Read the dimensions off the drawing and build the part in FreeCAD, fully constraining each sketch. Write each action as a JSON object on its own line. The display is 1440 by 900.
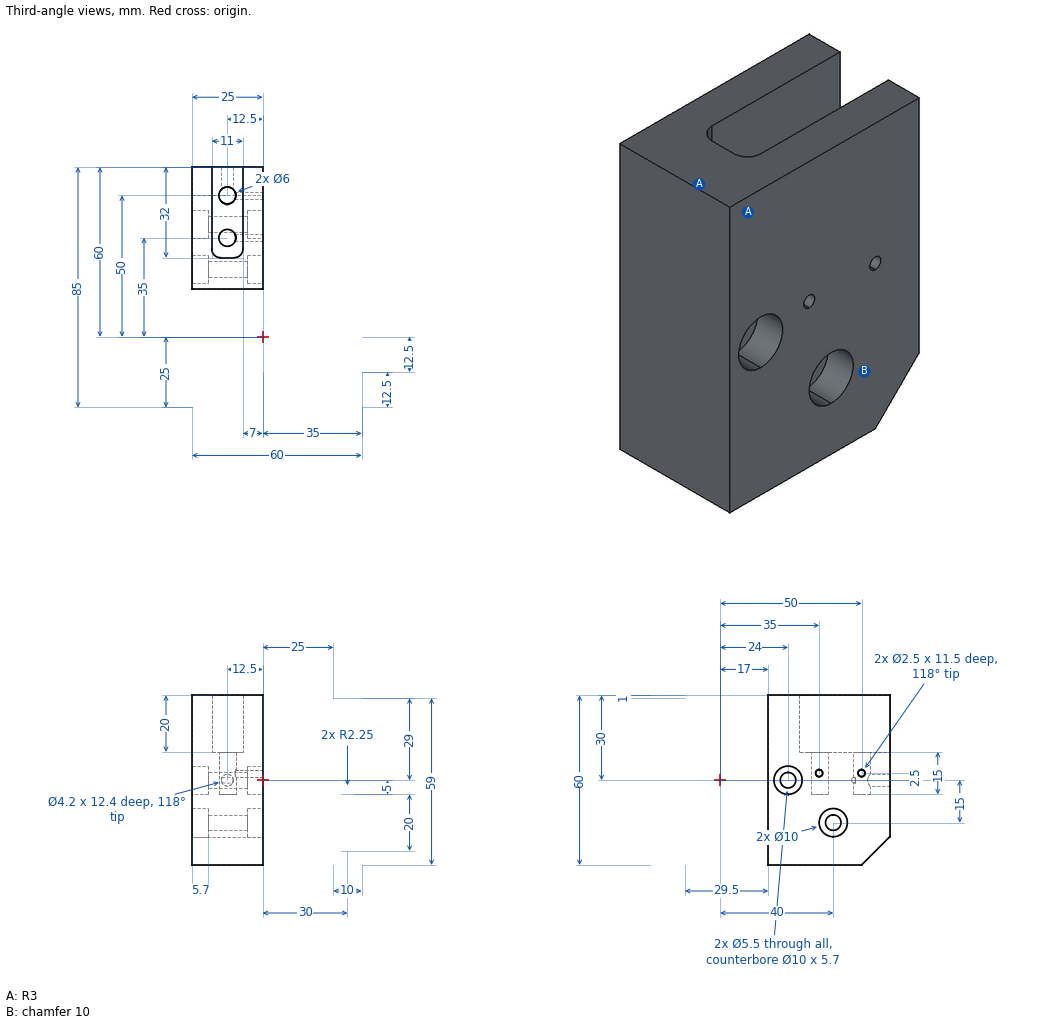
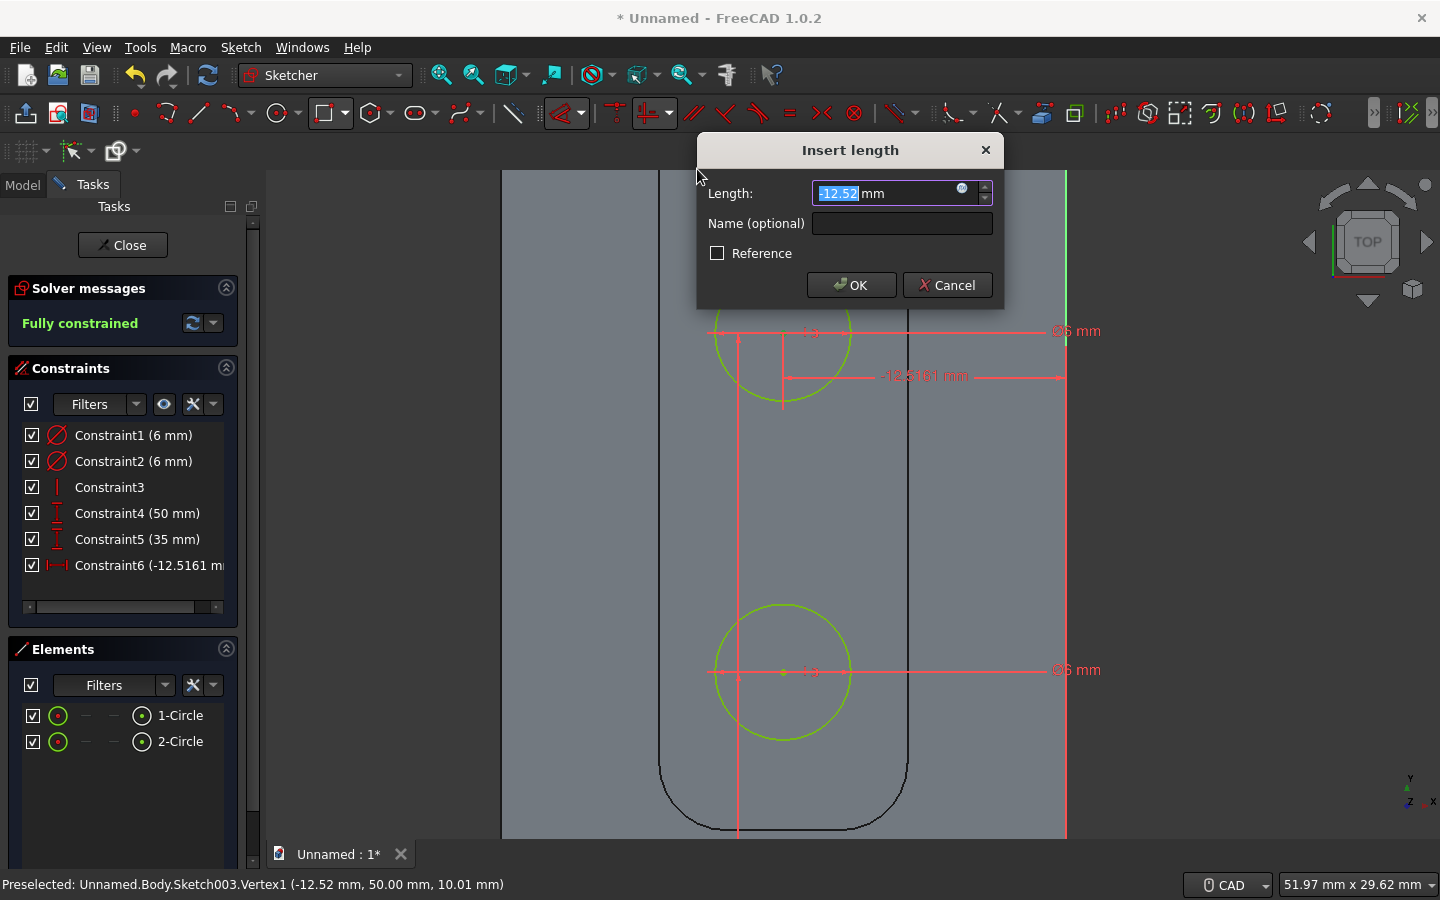
{"action": "type", "text": "-12.5"}
{"action": "key", "text": "Return"}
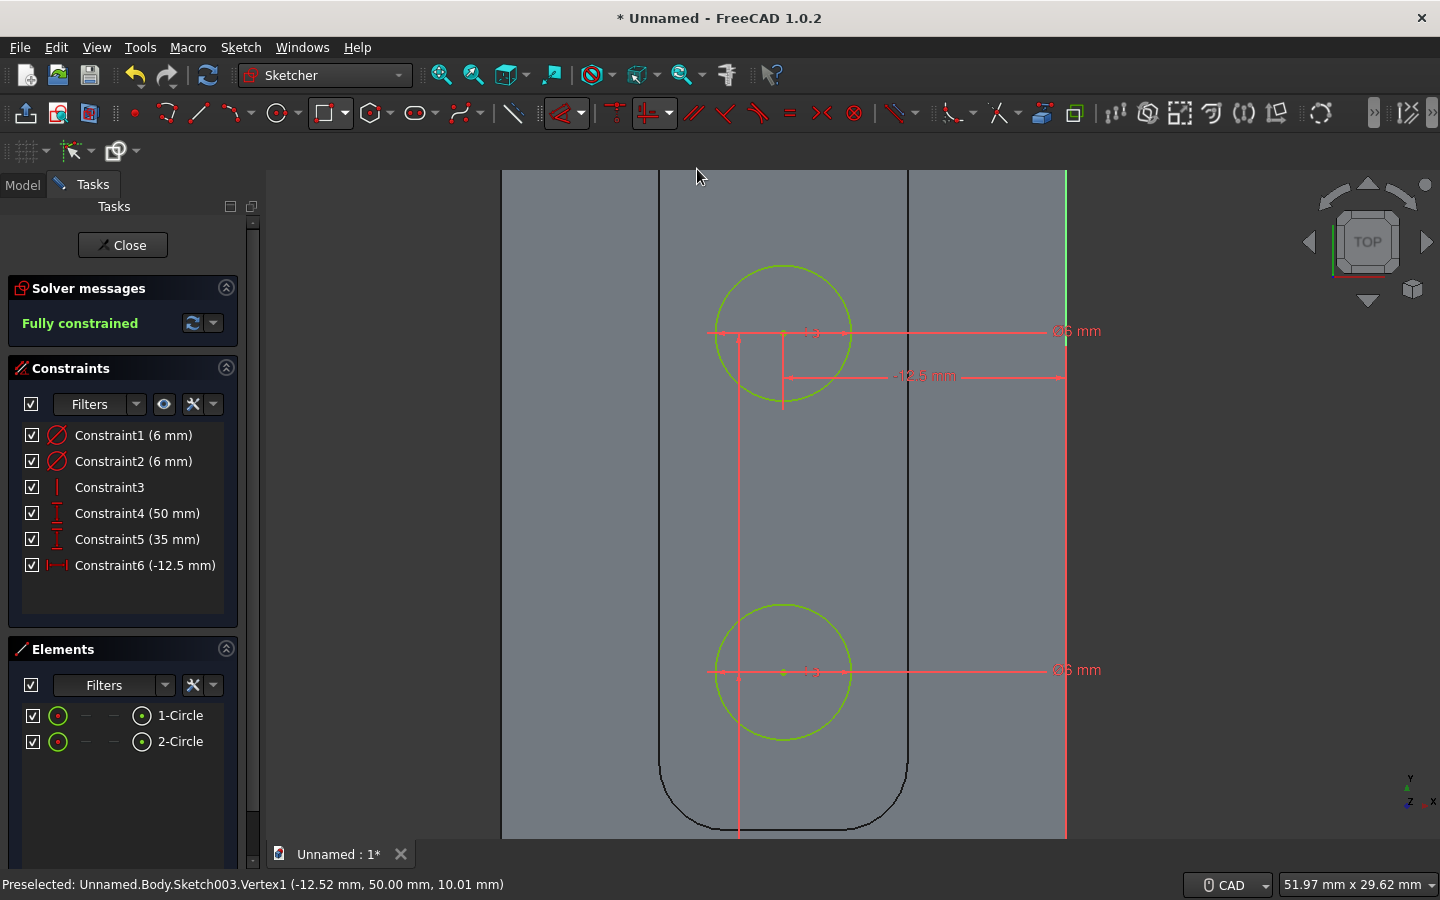
{"action": "left_click", "coordinate": [123, 245]}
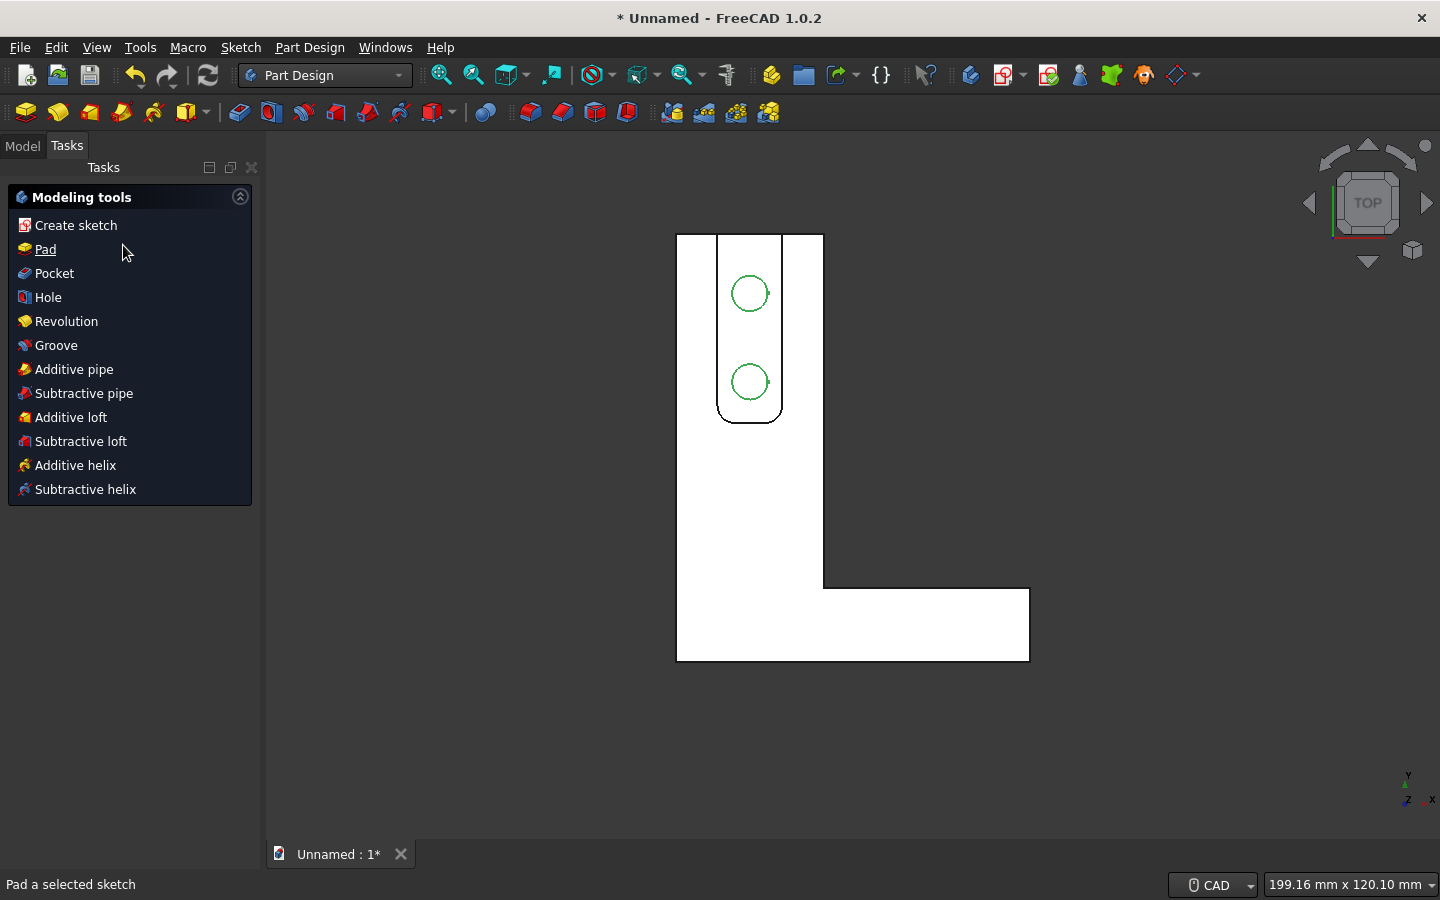
{"action": "left_click", "coordinate": [240, 112]}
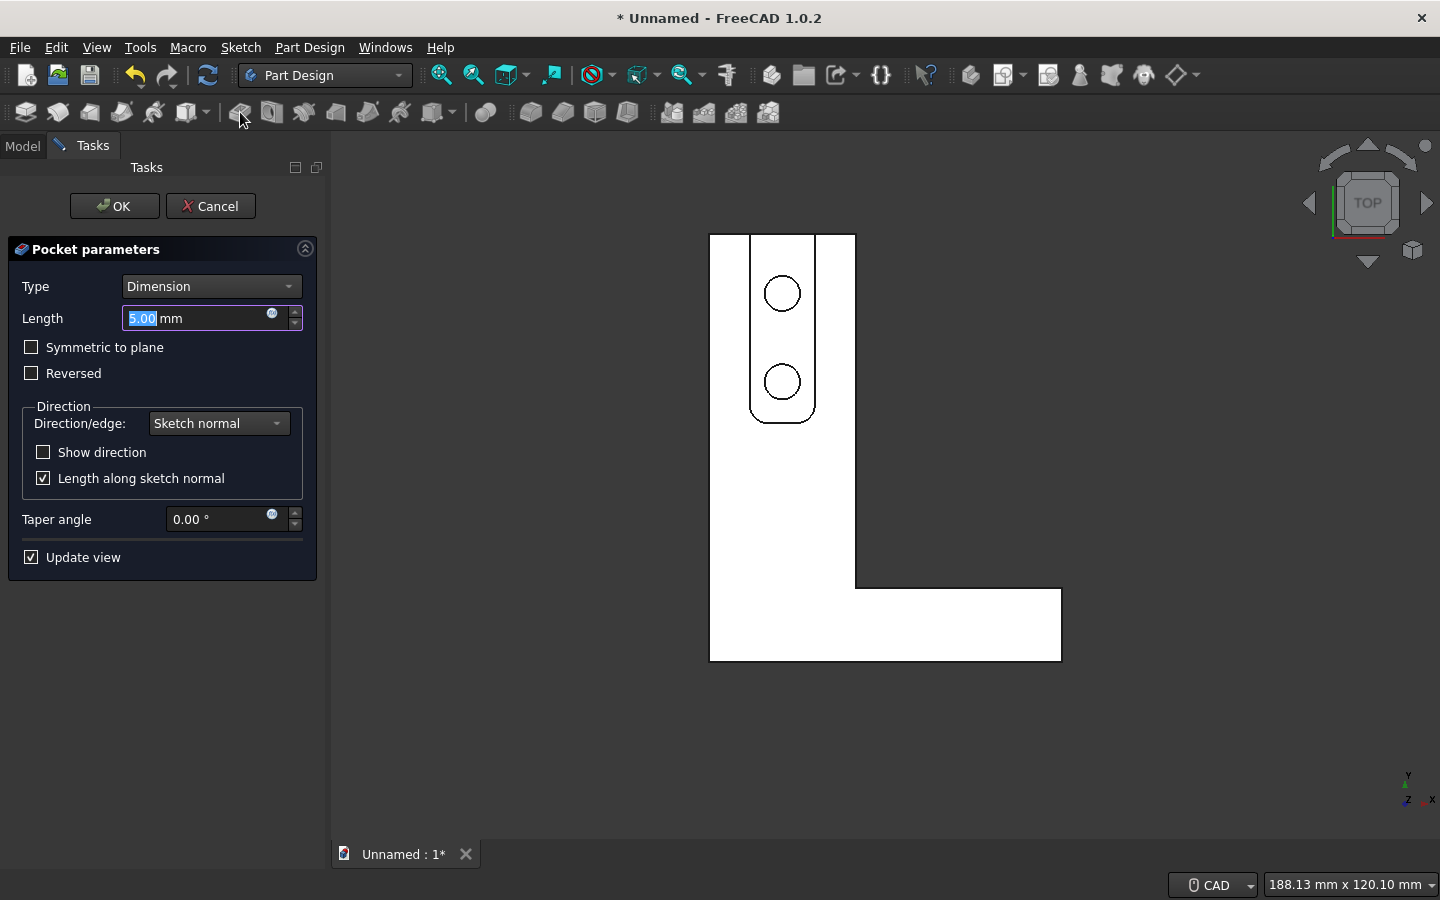
{"action": "type", "text": "15"}
{"action": "key", "text": "Tab"}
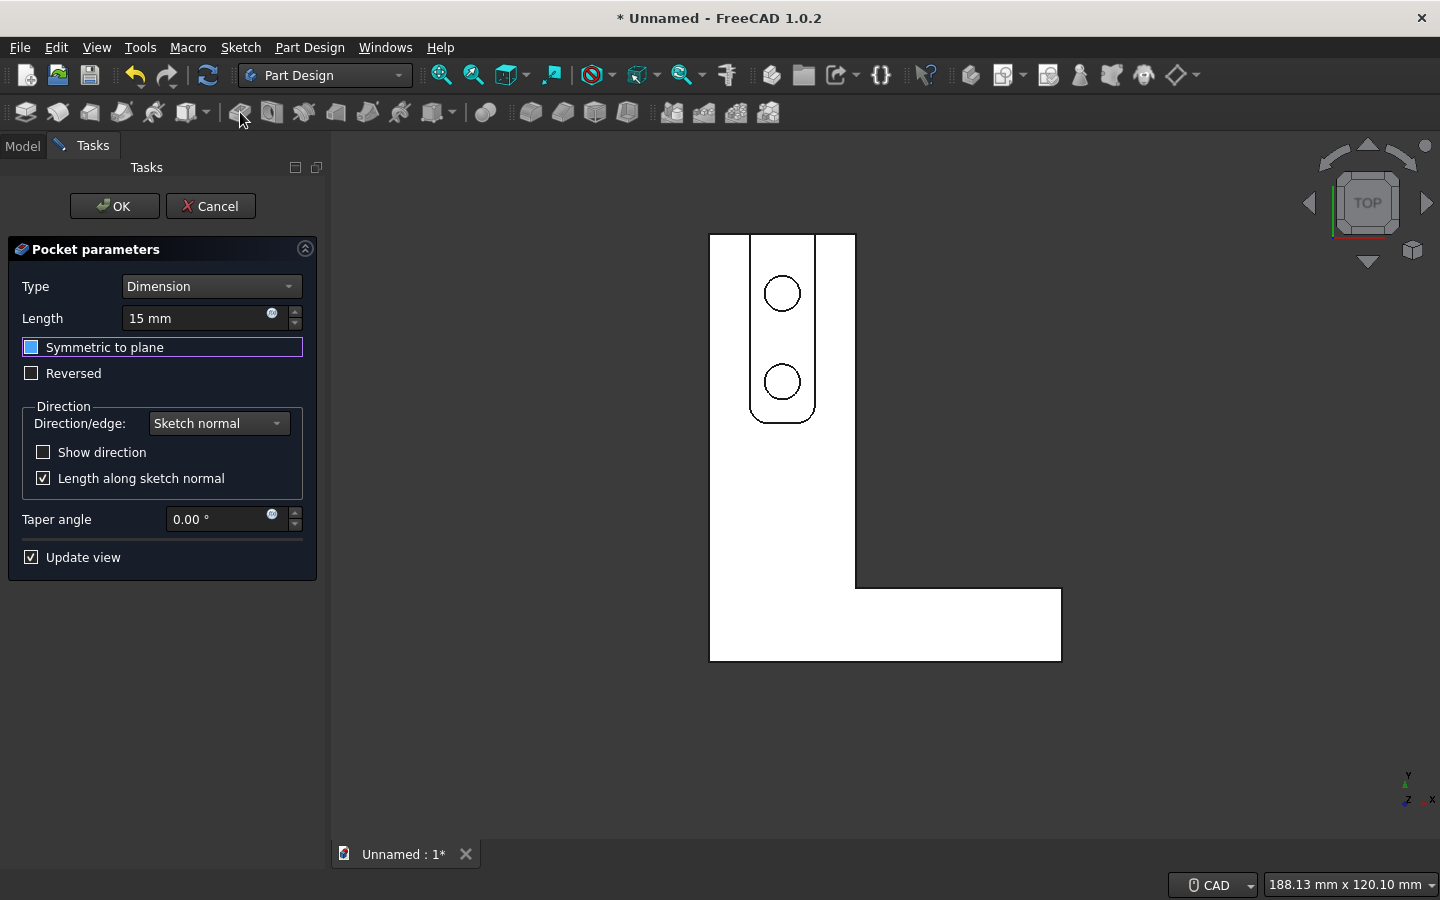
{"action": "left_click", "coordinate": [115, 206]}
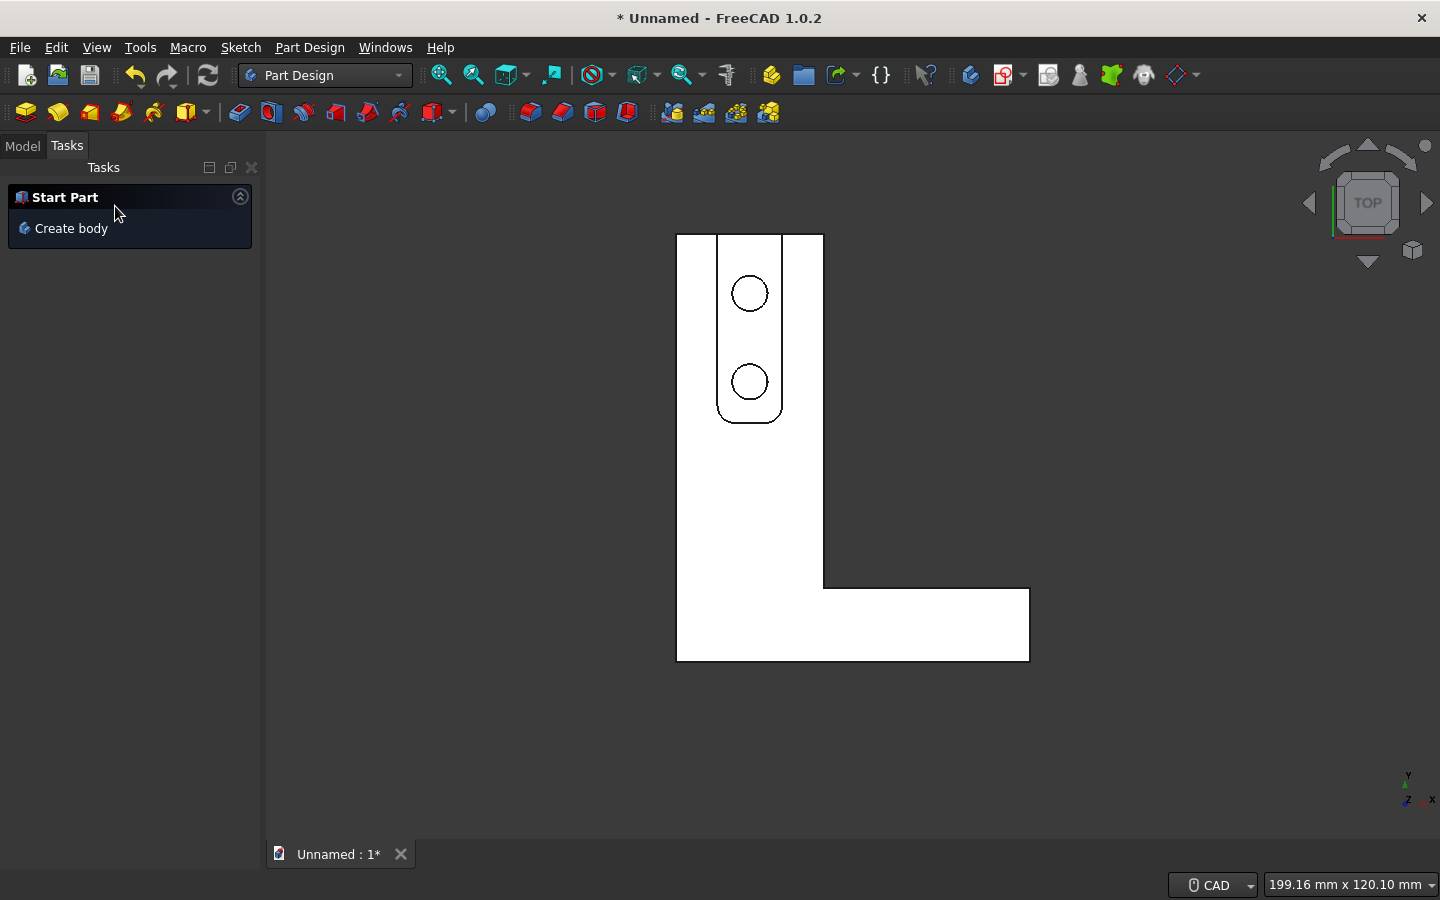
{"action": "key", "text": "0"}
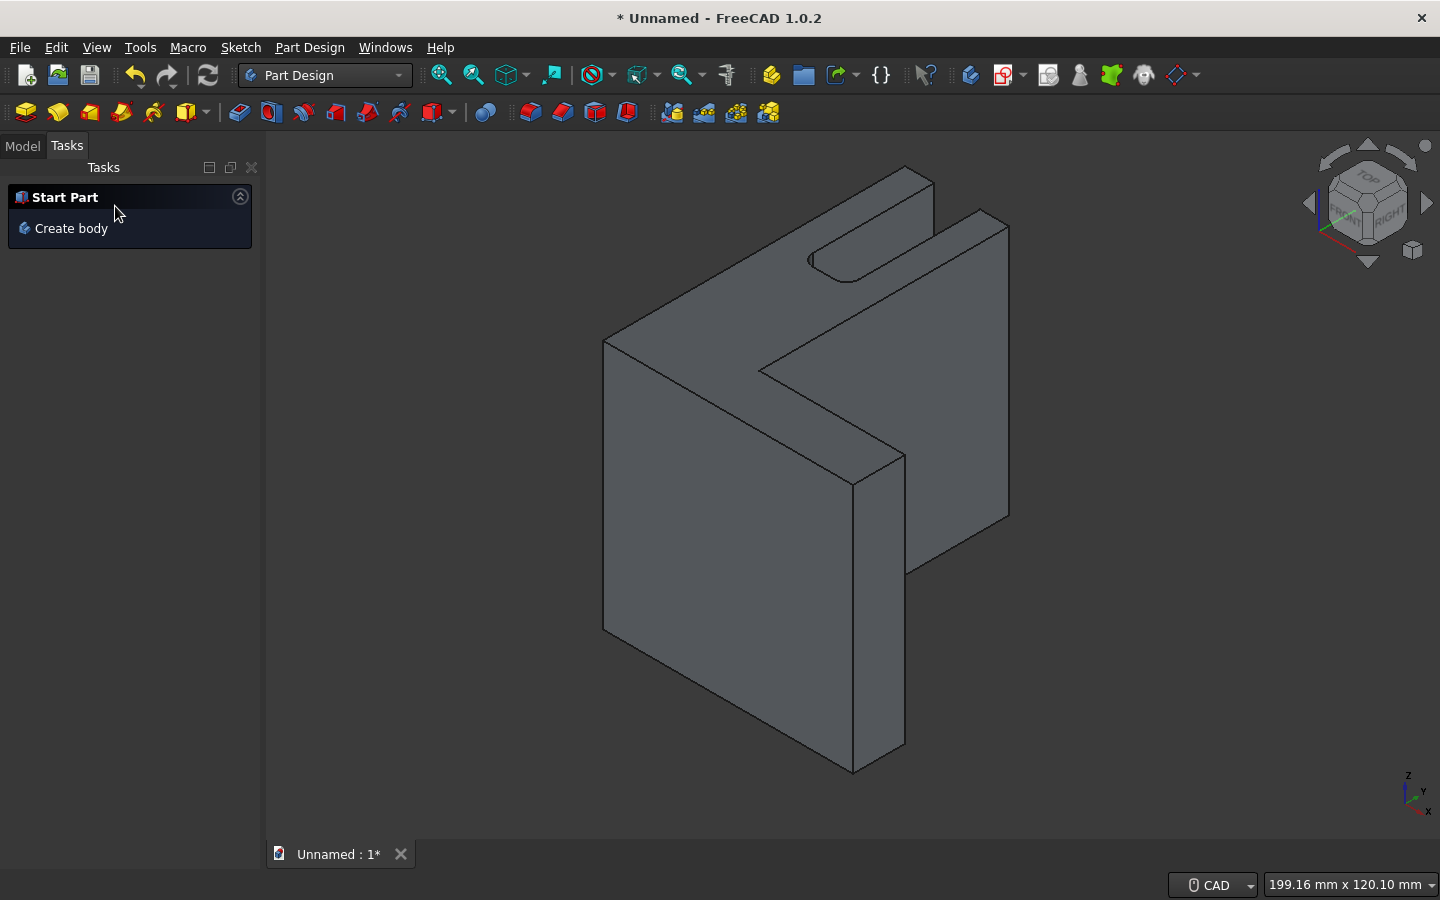
{"action": "left_click", "coordinate": [920, 380]}